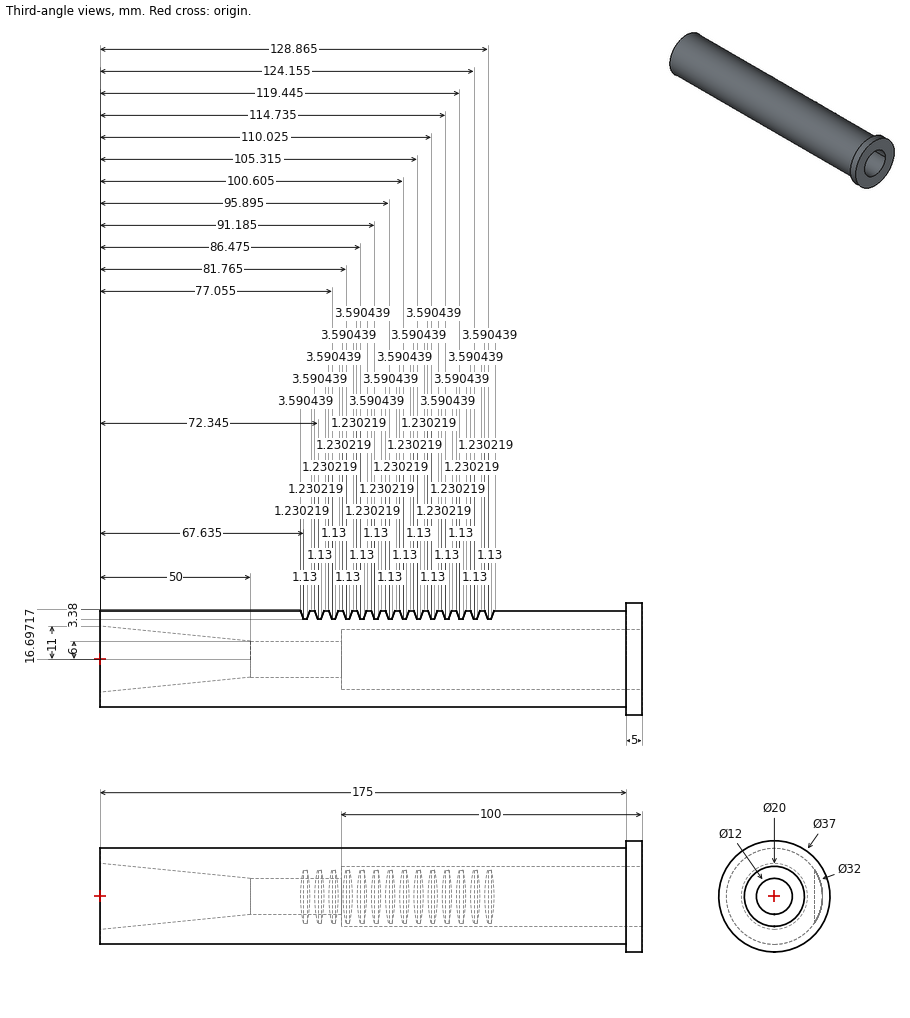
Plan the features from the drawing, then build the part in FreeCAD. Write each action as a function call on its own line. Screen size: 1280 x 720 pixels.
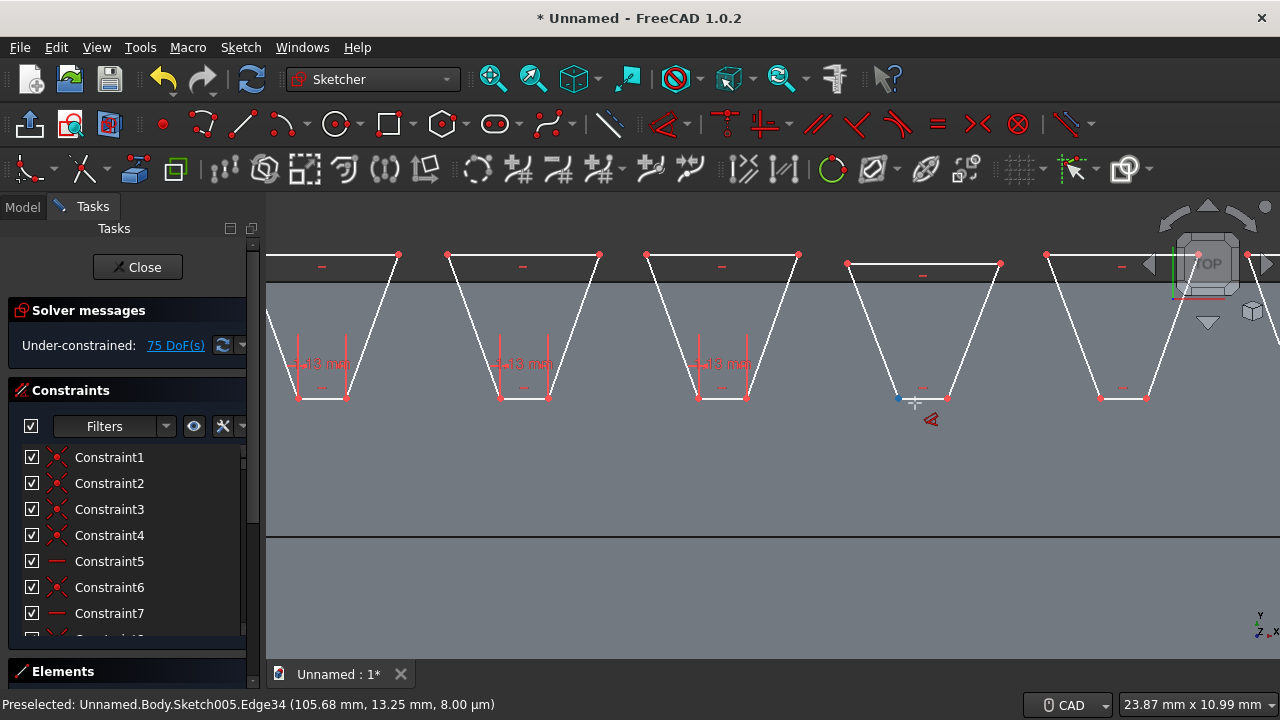
click(914, 399)
click(923, 365)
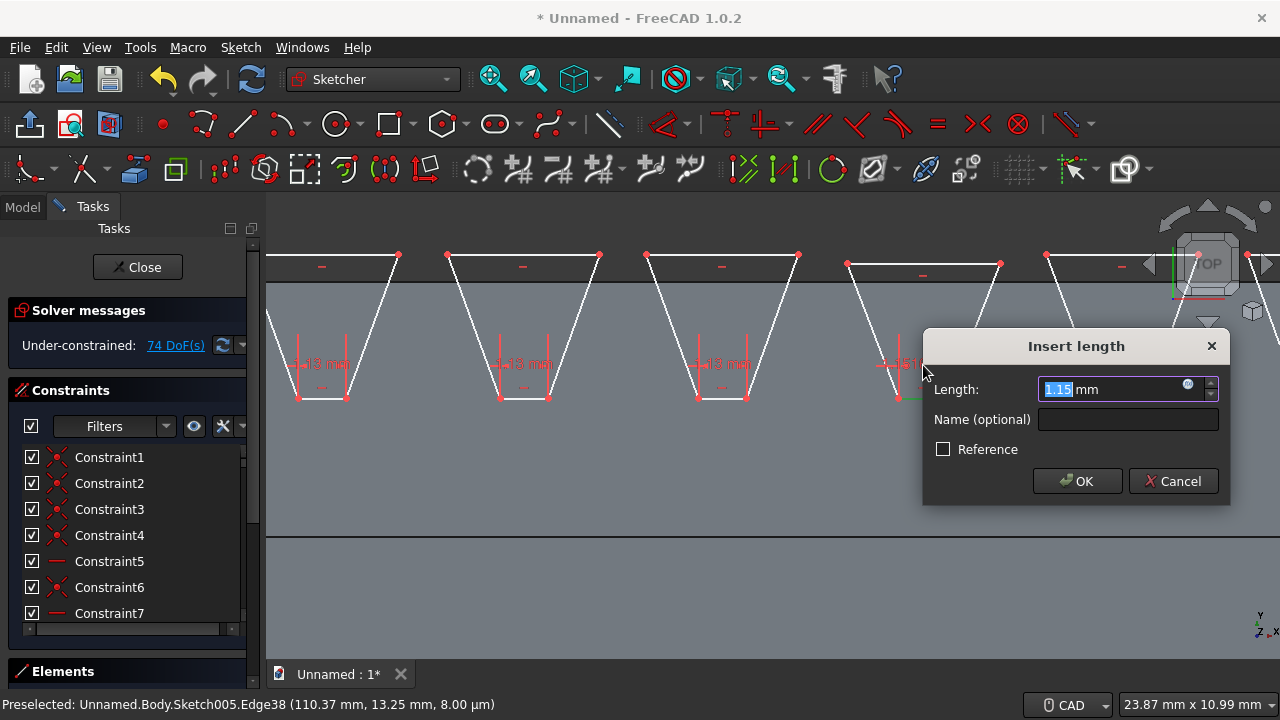
text(1.13)
key(Return)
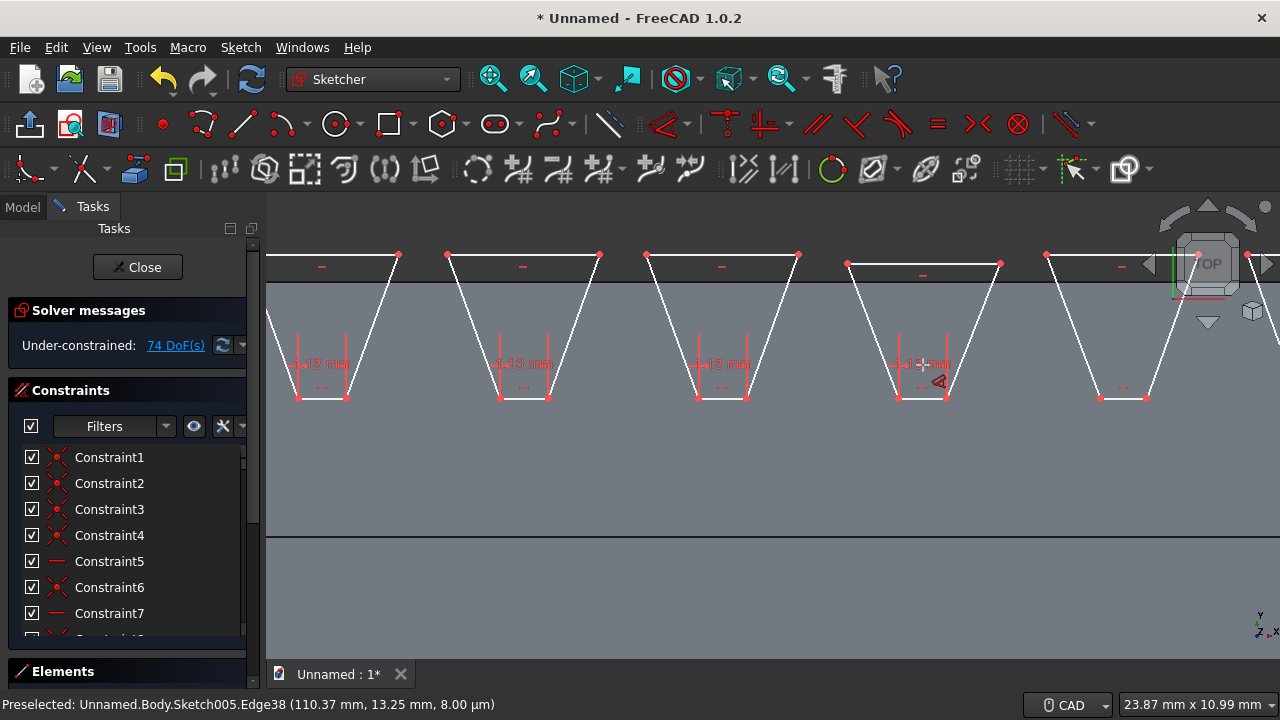
click(1115, 399)
click(1108, 365)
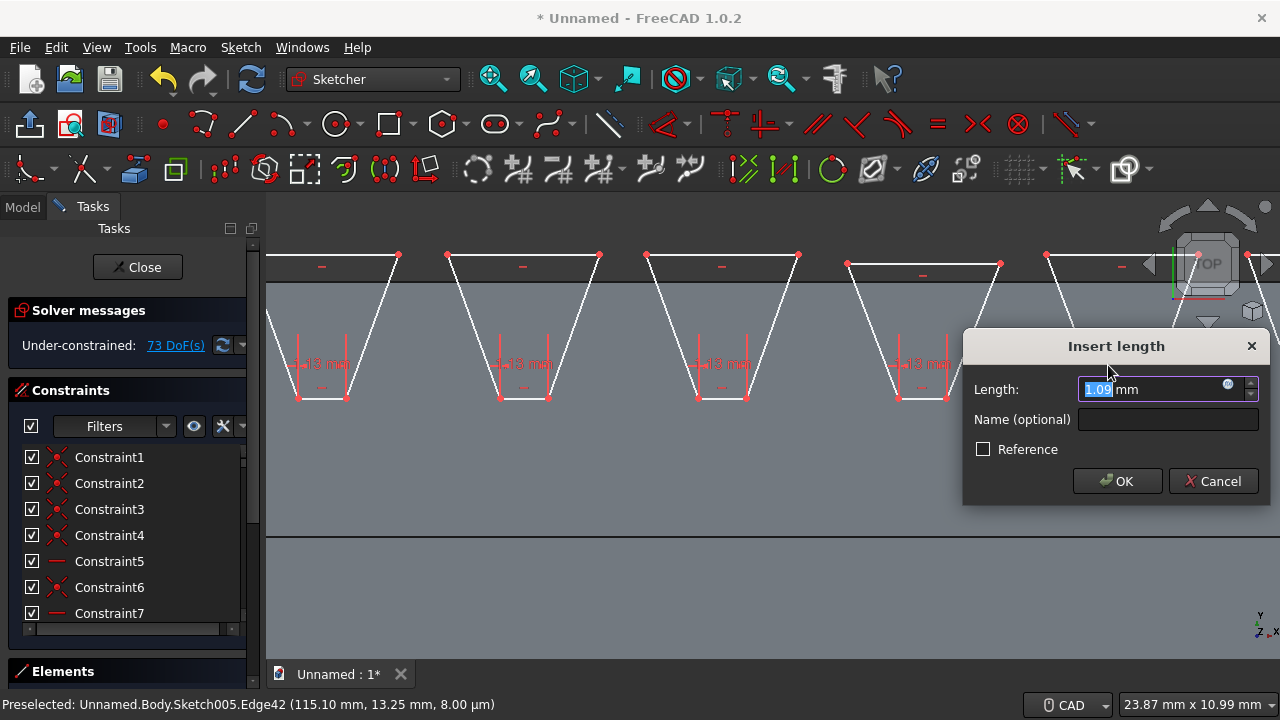
text(1.13)
key(Return)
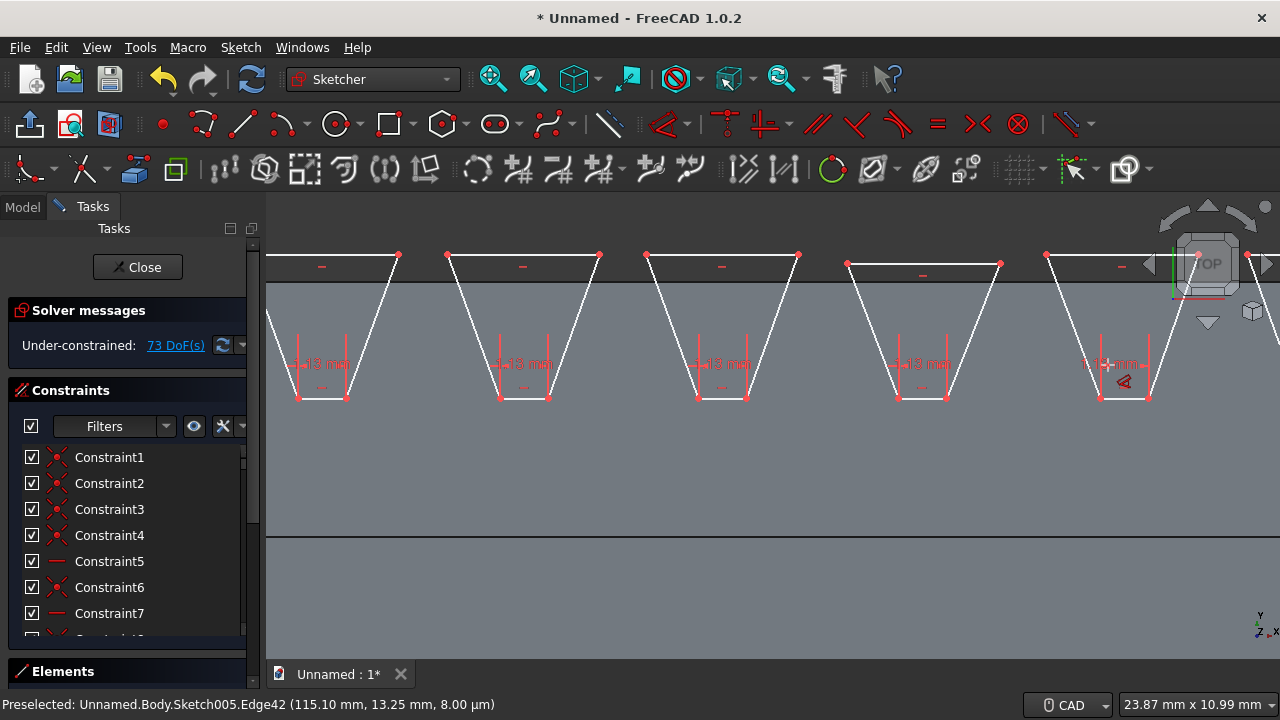
scroll(915, 403, down, 11)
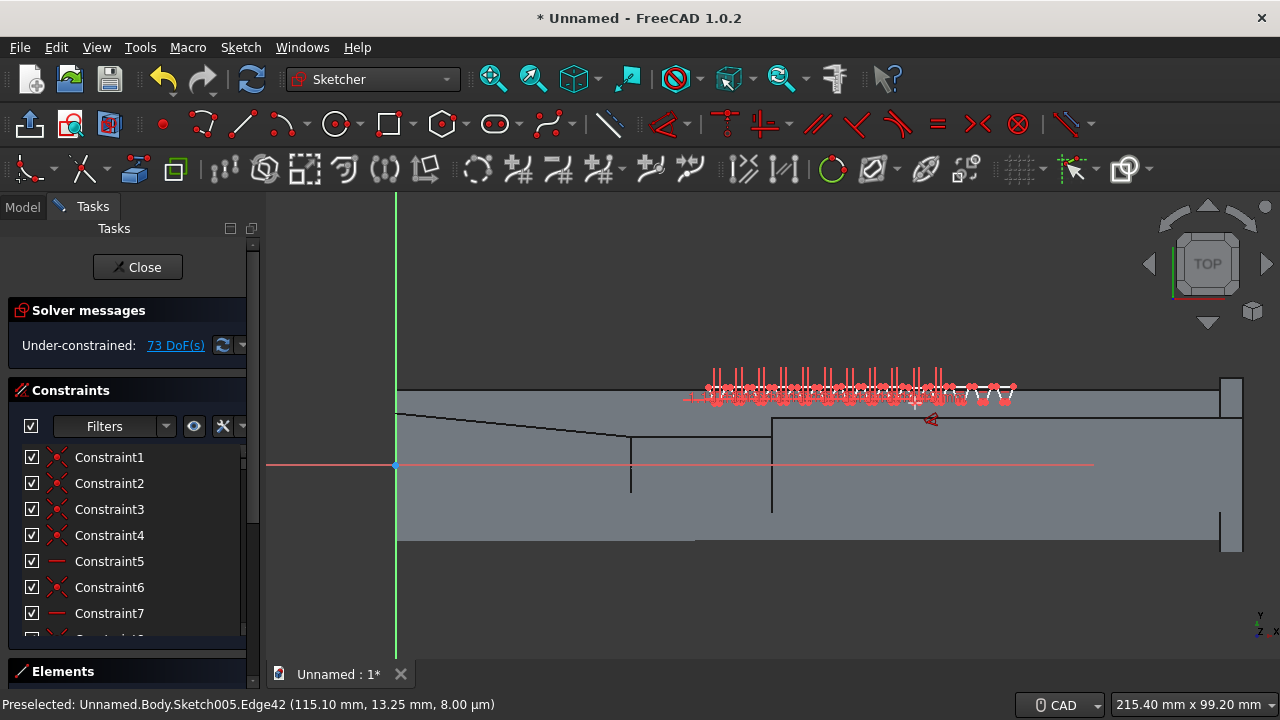
scroll(960, 403, up, 11)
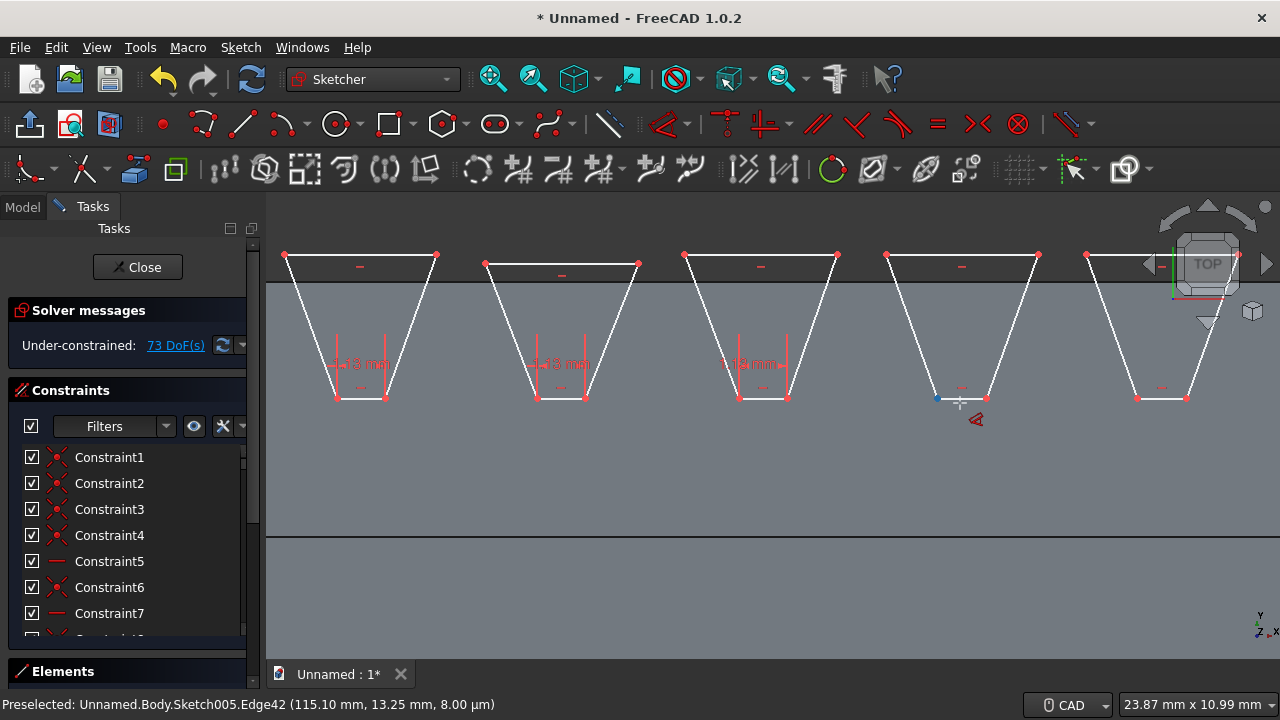
click(952, 399)
click(962, 365)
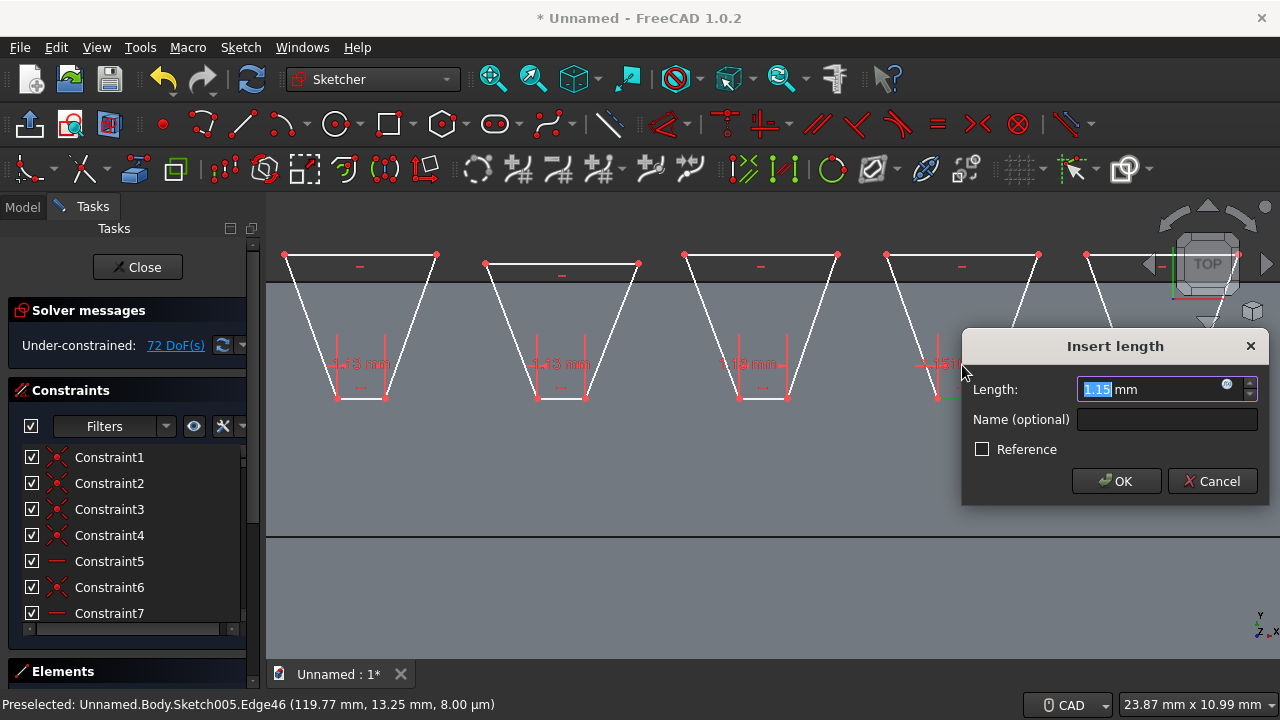
text(1.13)
key(Return)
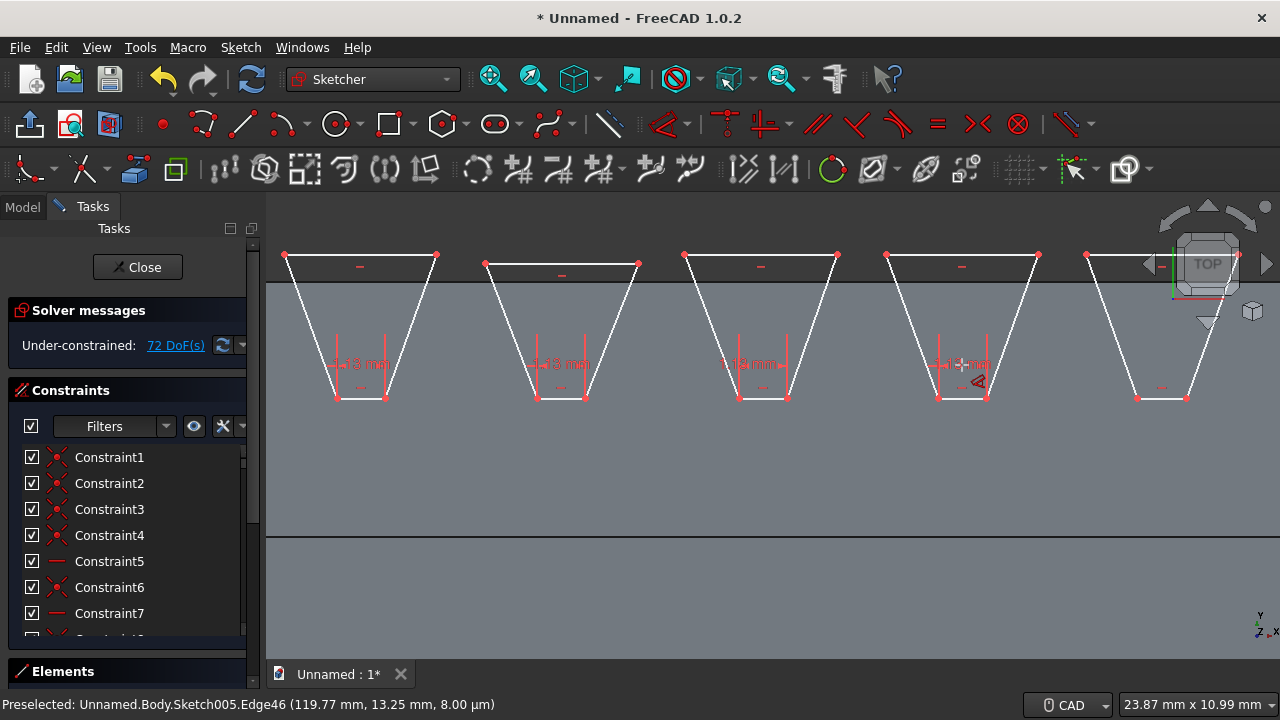
scroll(960, 403, down, 11)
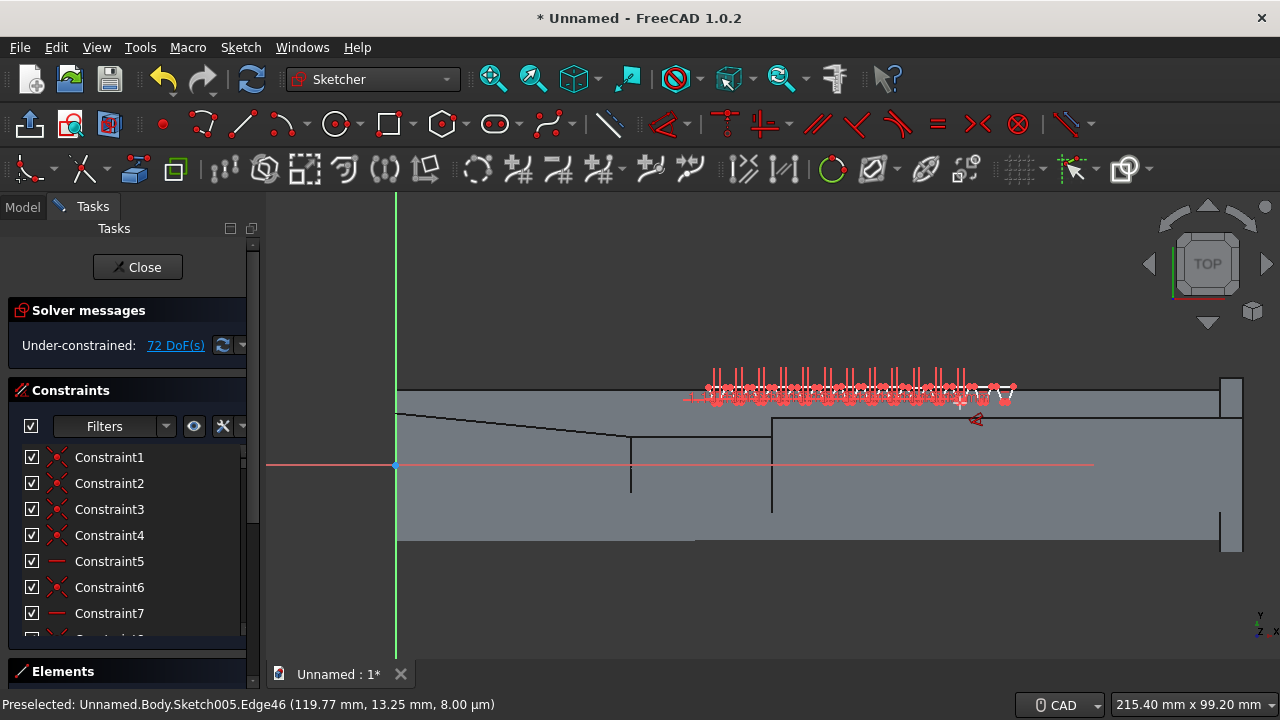
scroll(982, 403, up, 11)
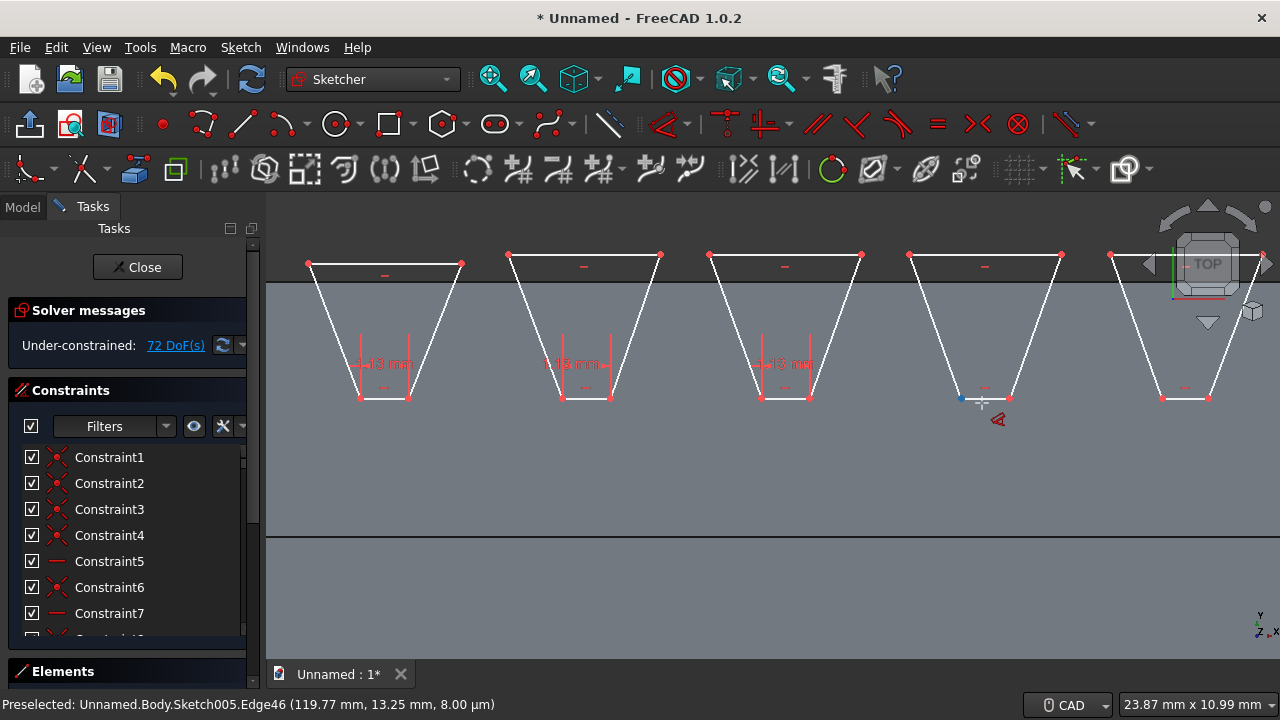
click(976, 399)
click(986, 365)